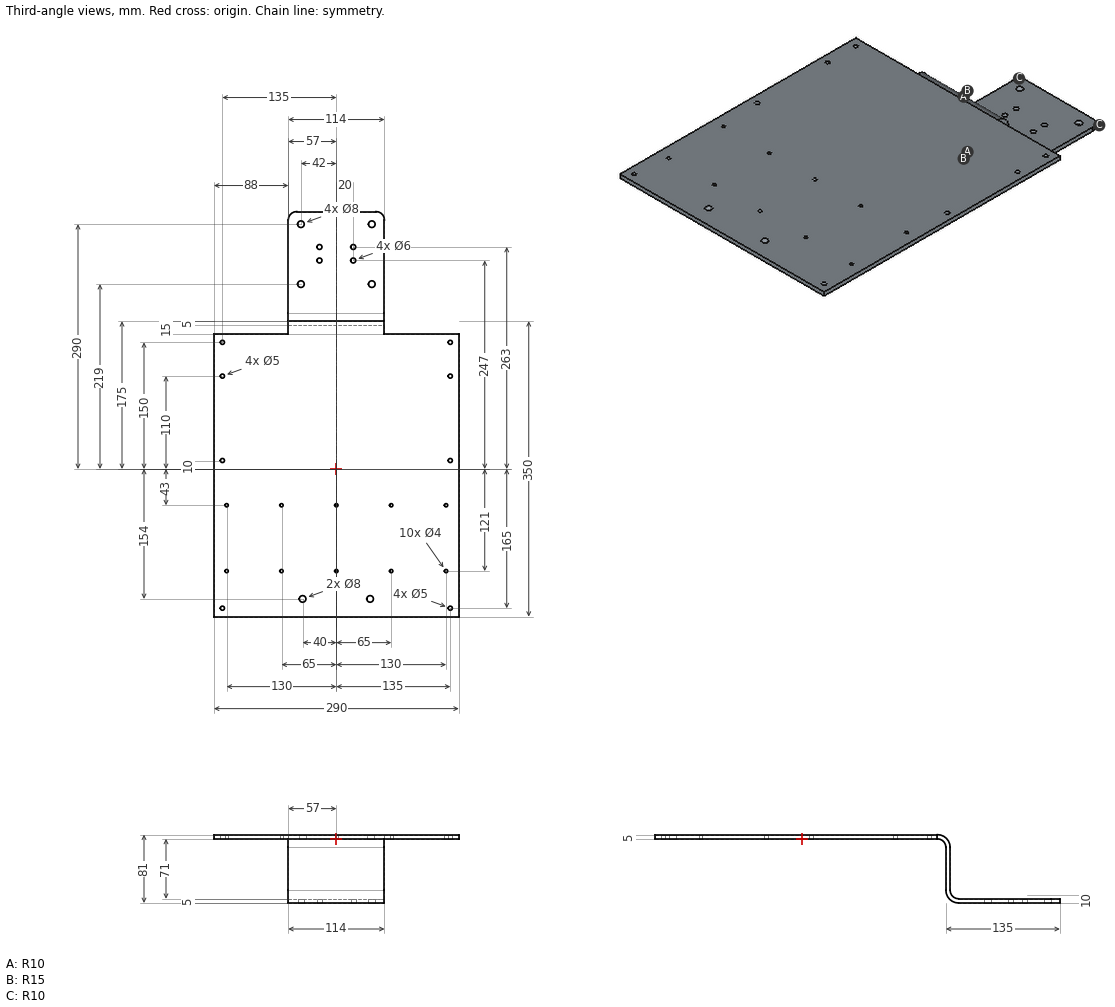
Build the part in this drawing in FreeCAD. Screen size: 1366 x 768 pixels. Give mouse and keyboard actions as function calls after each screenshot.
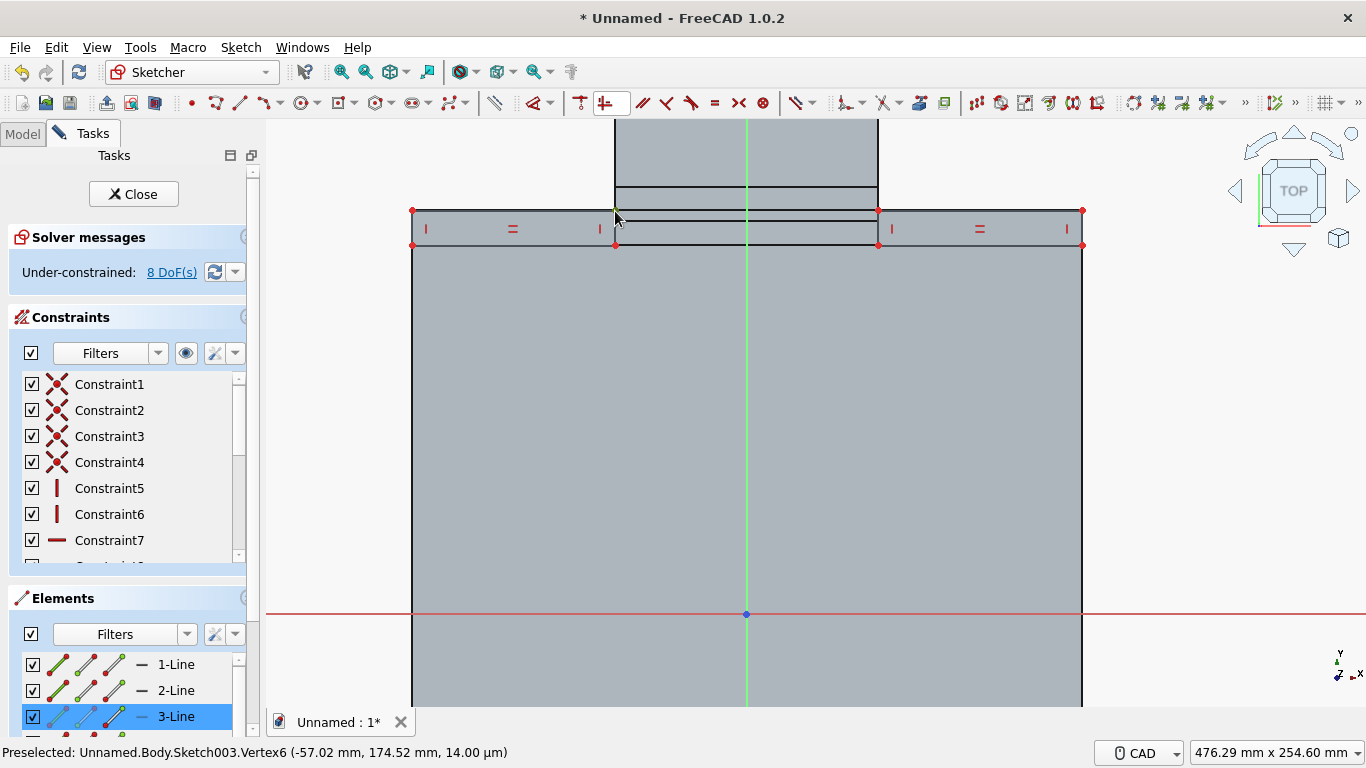
click(878, 211)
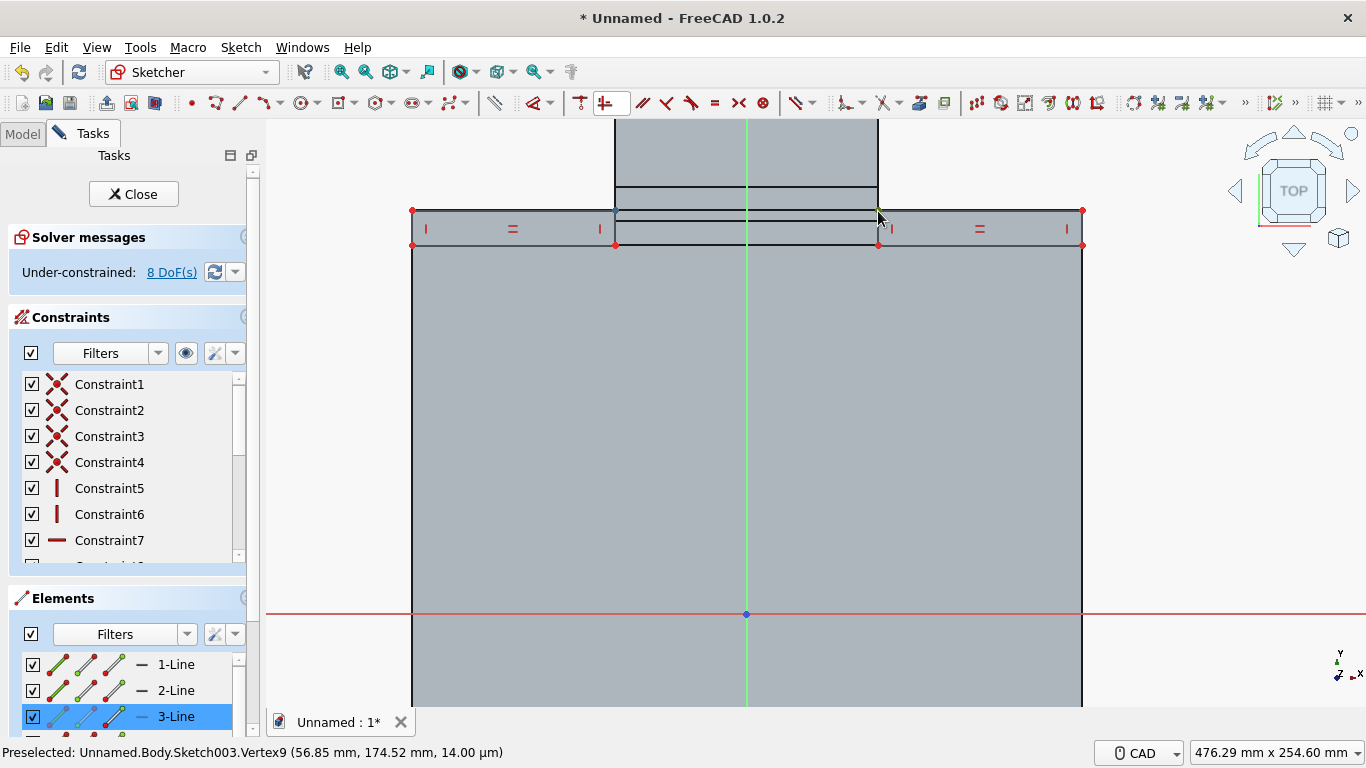
click(747, 565)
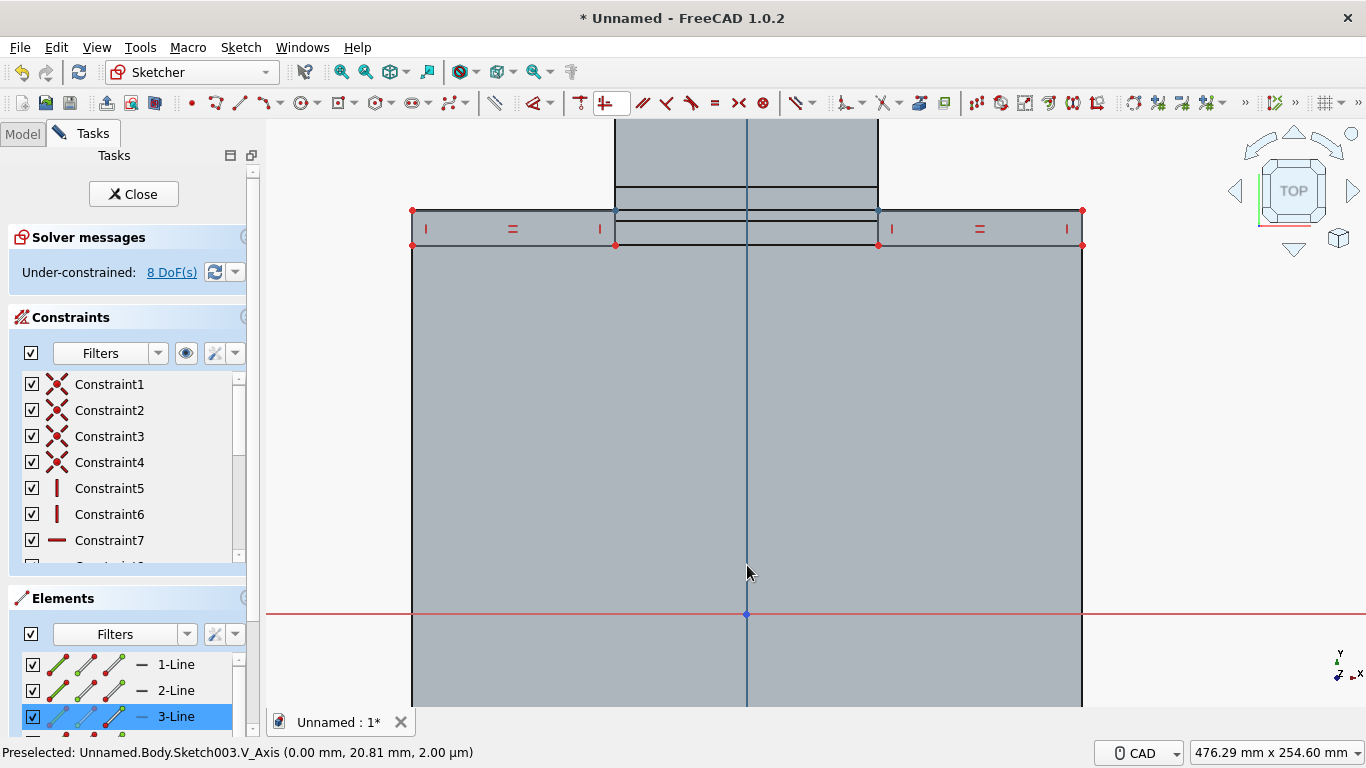
click(740, 104)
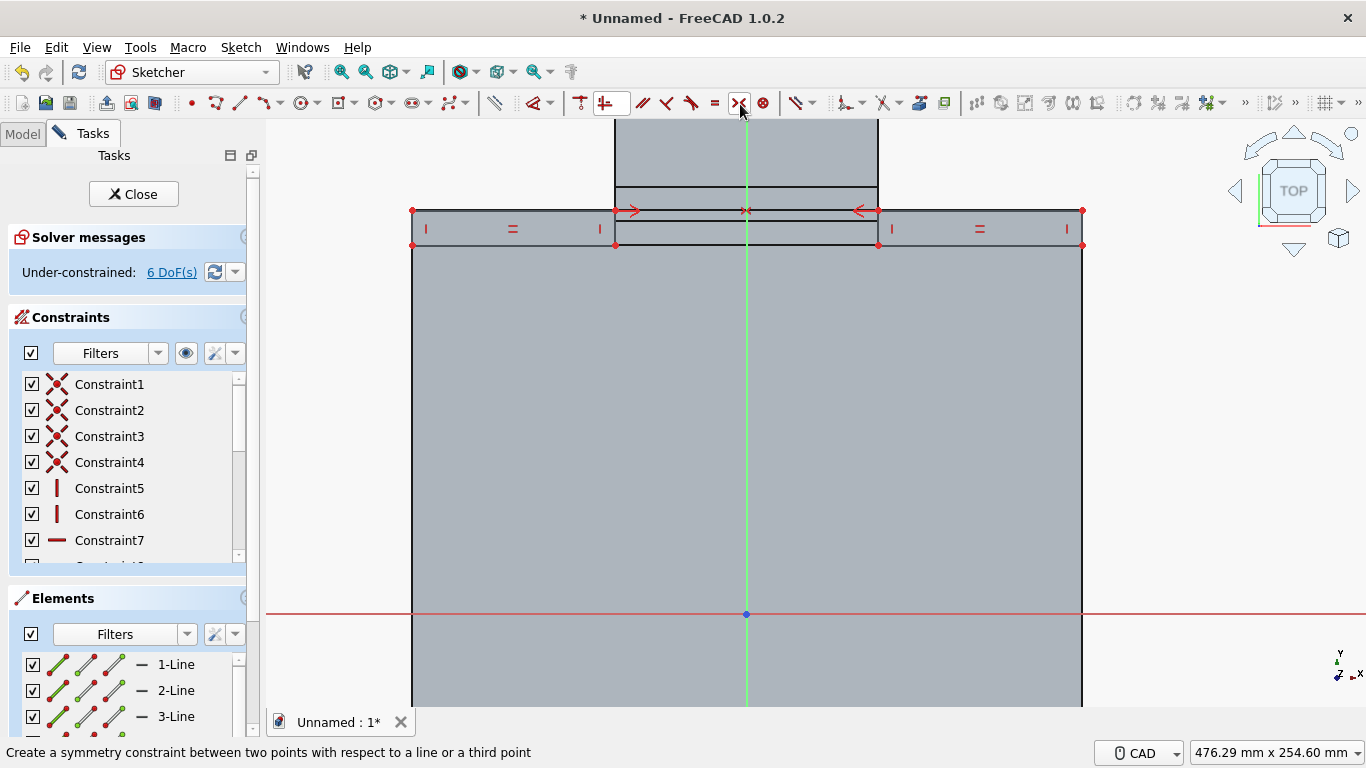
click(412, 246)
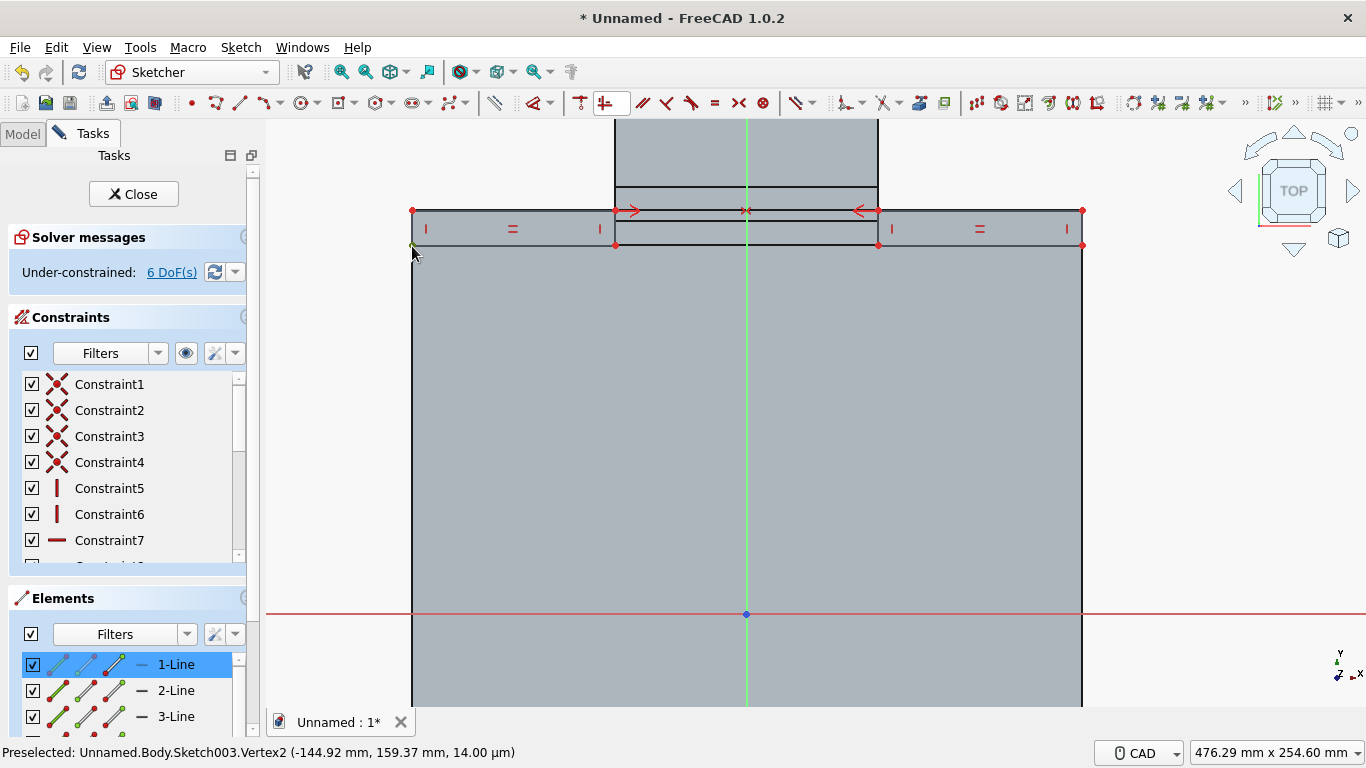
click(1082, 246)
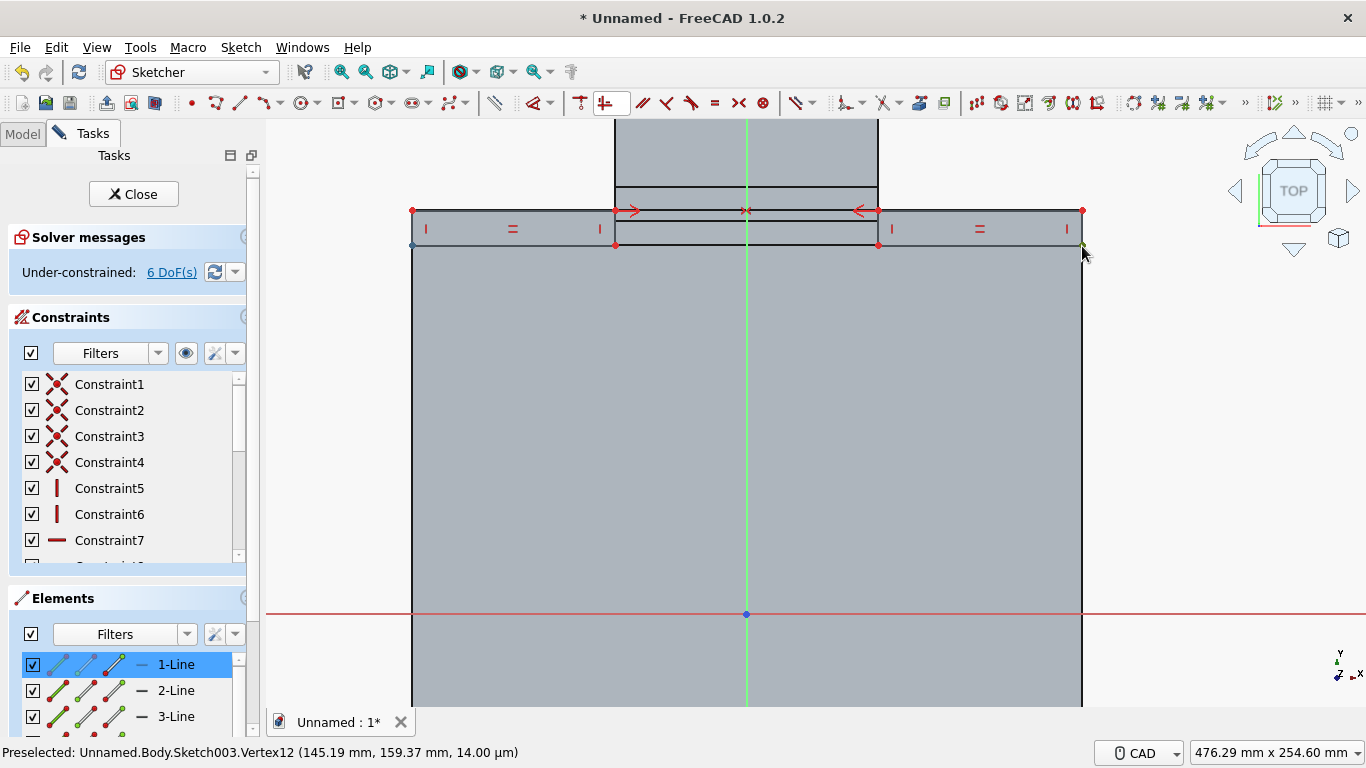
click(747, 565)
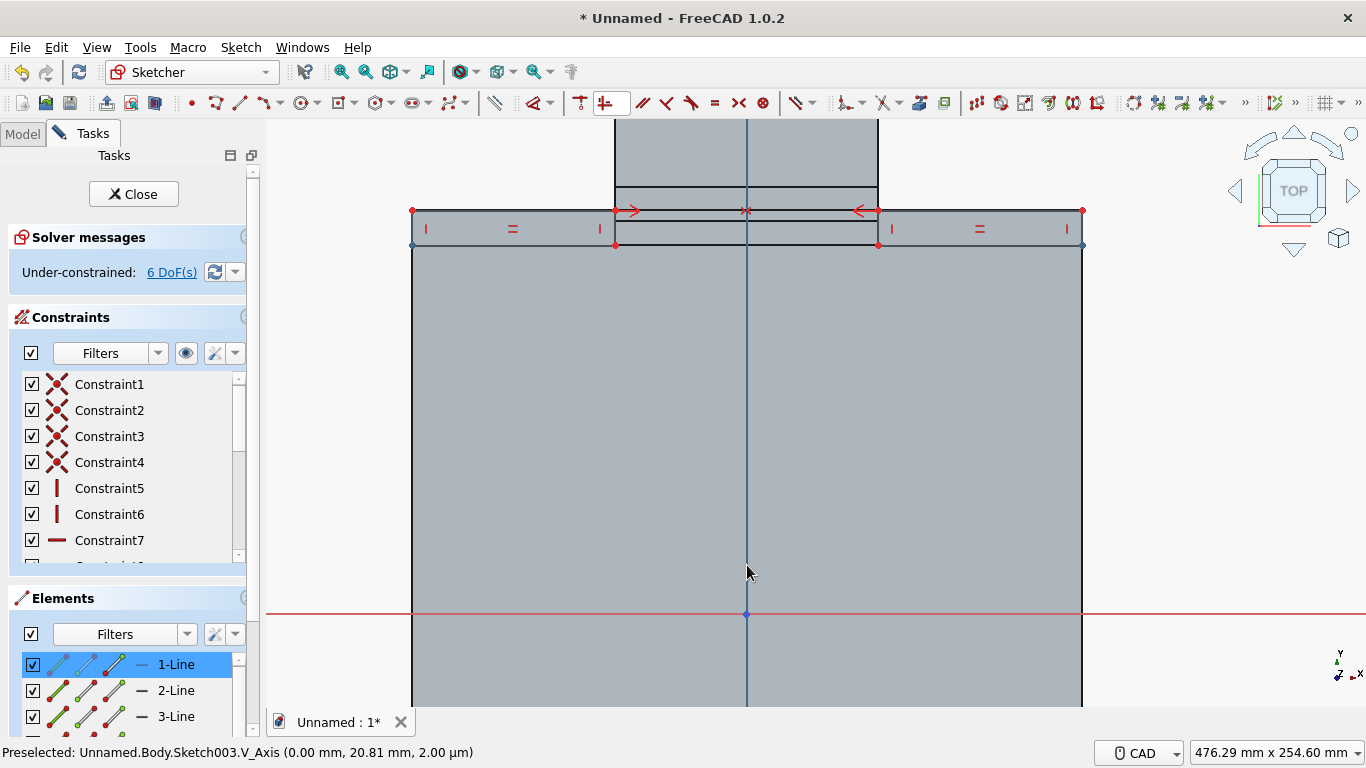
click(740, 104)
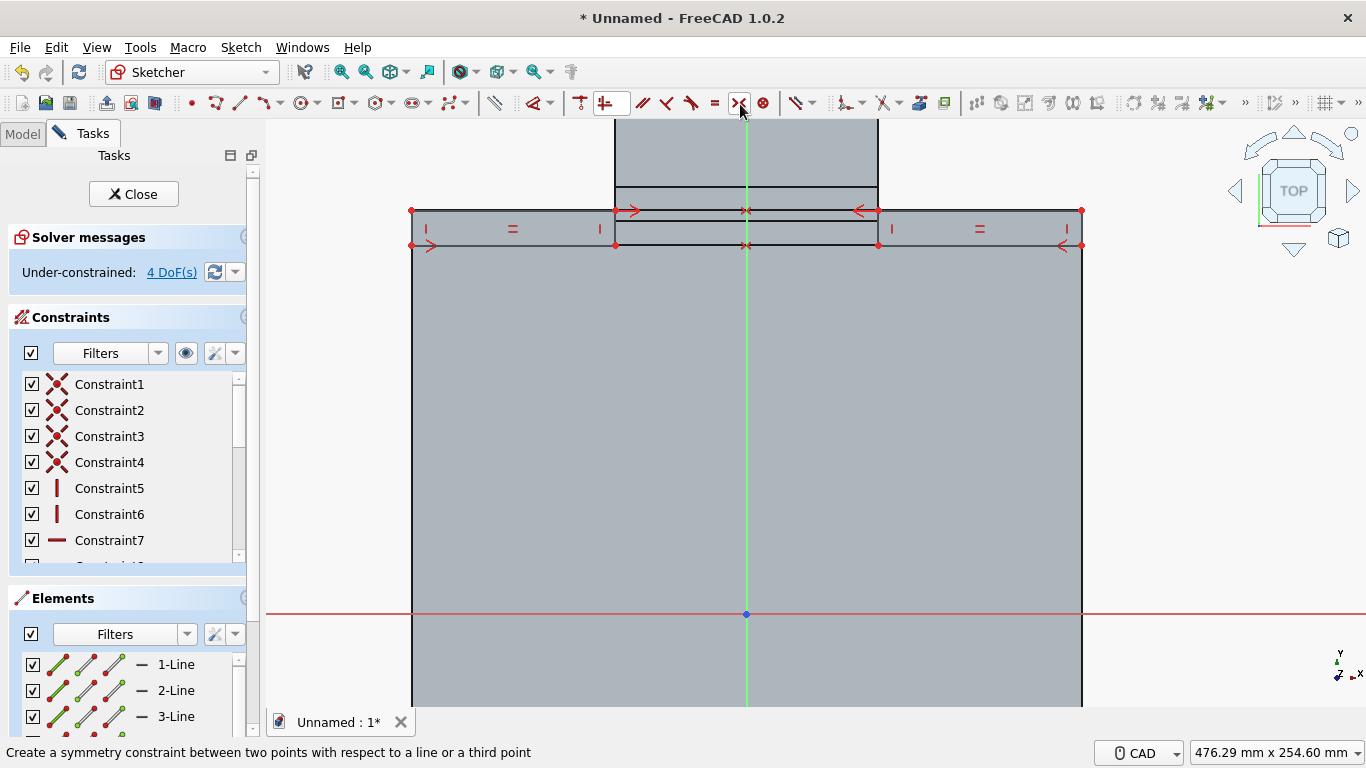
click(534, 104)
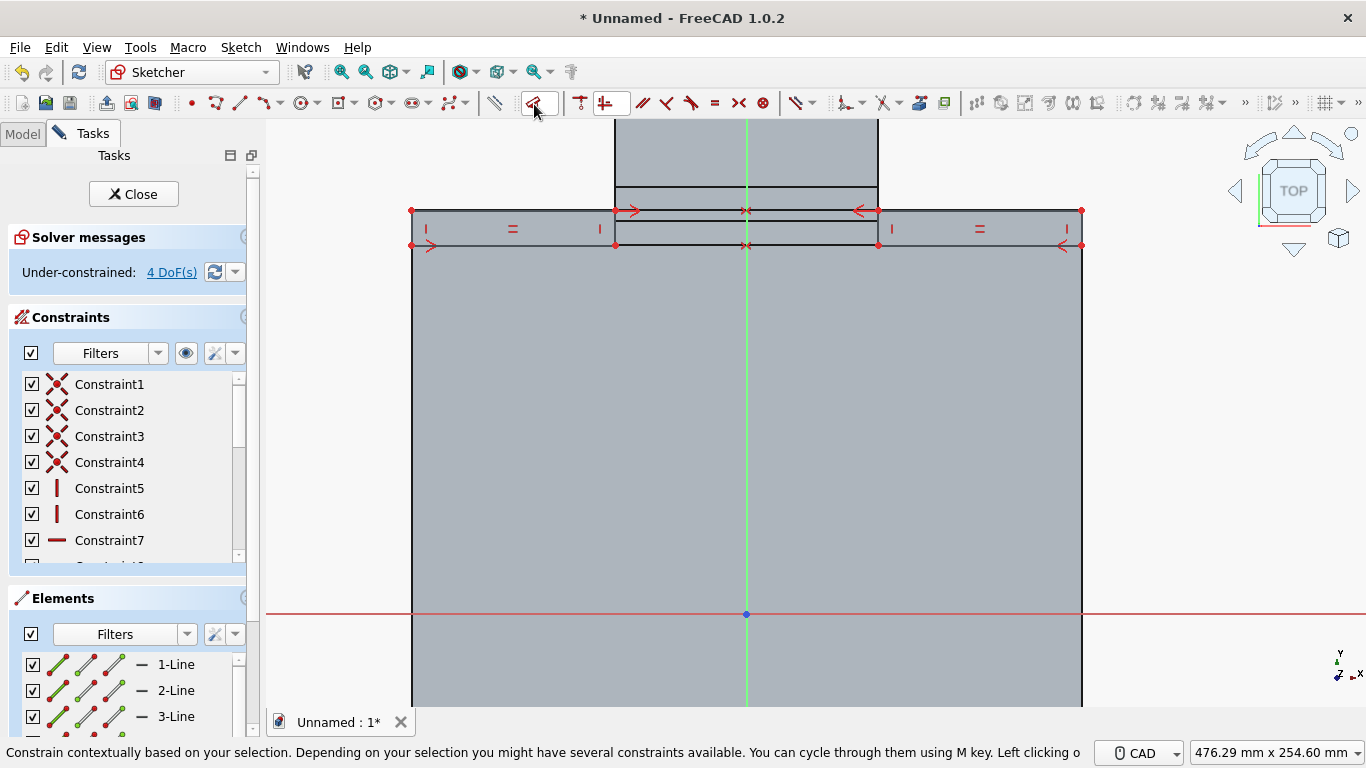
scroll(412, 222, up, 2)